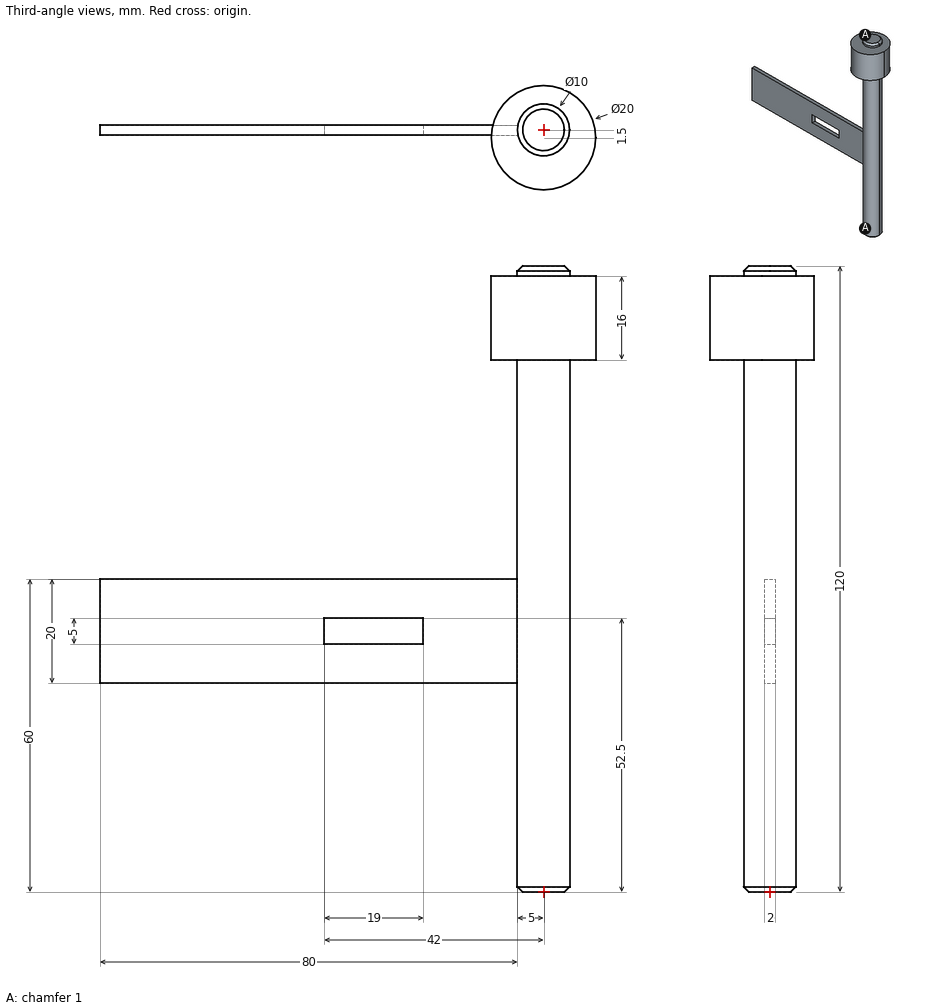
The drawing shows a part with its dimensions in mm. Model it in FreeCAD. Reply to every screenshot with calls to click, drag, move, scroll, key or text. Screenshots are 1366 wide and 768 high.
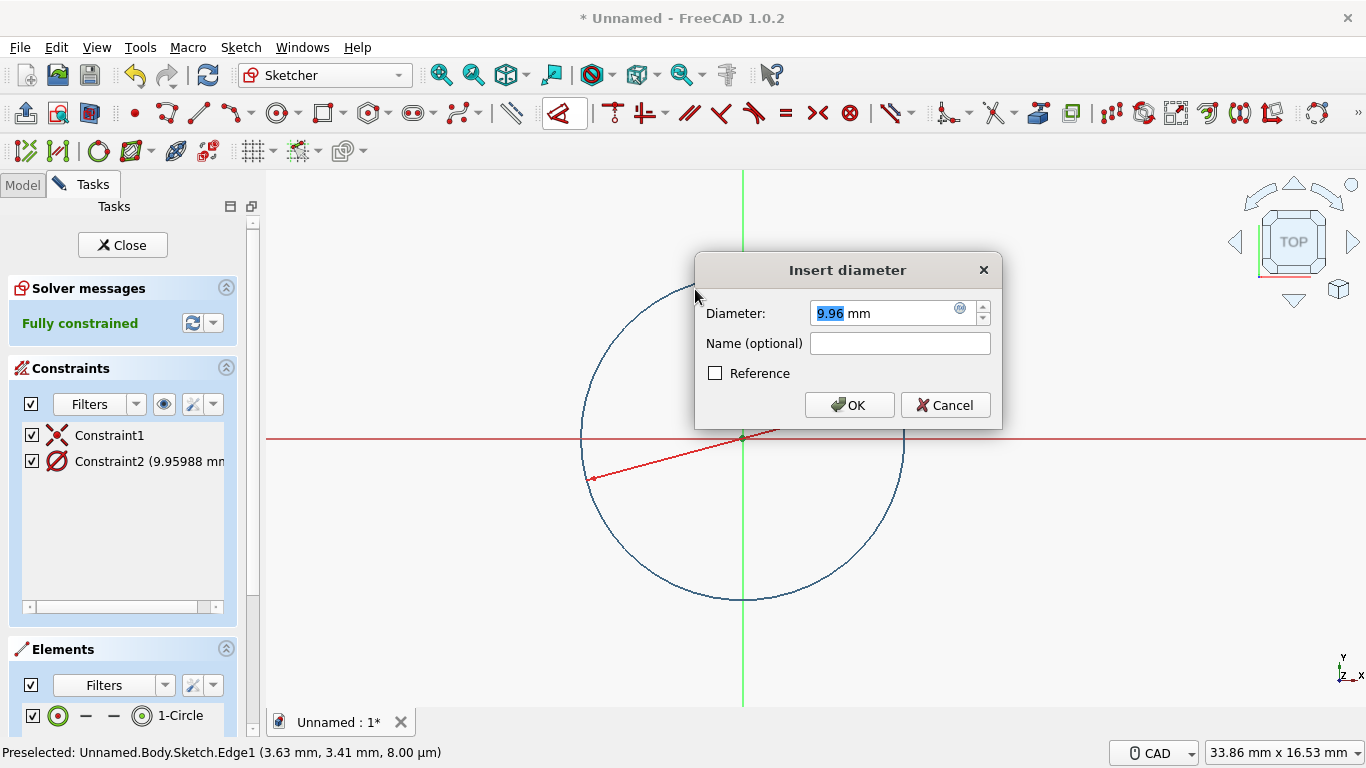
text(10)
key(Return)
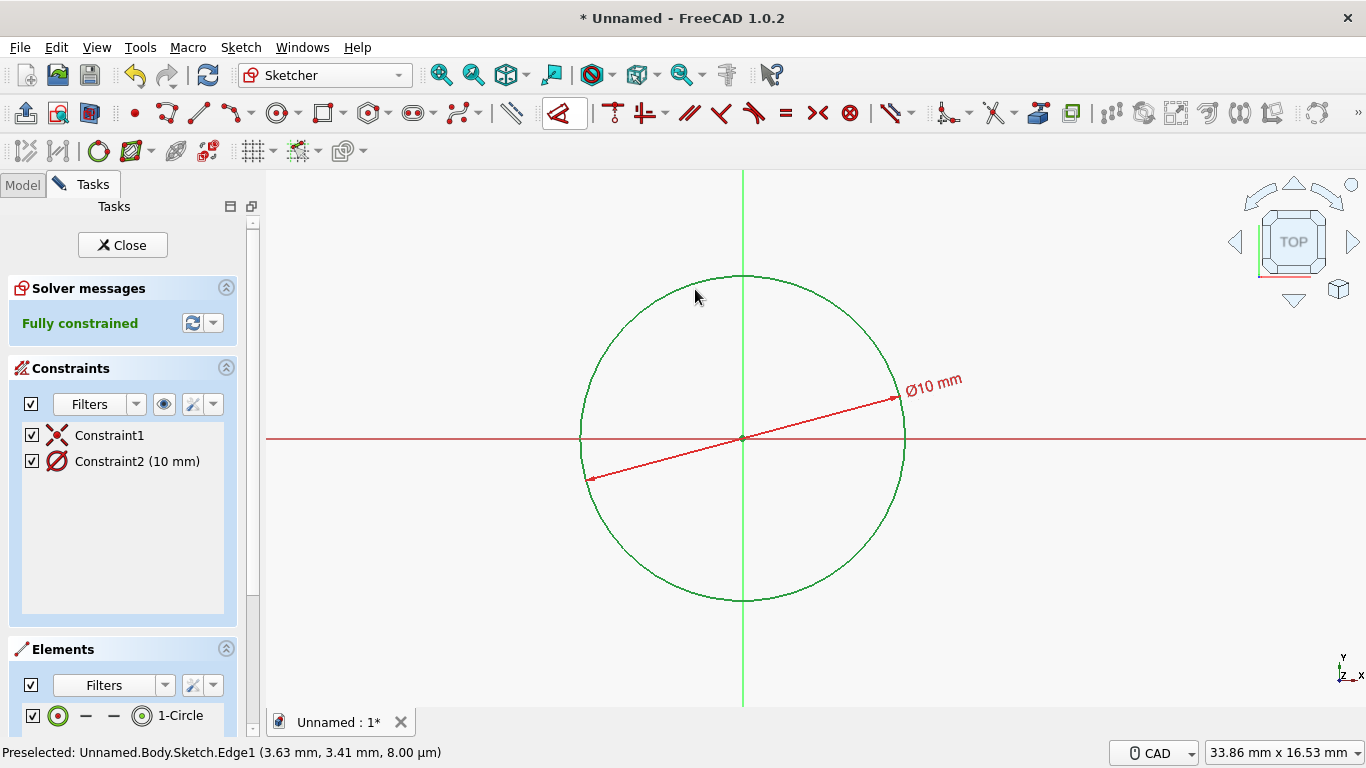
click(123, 245)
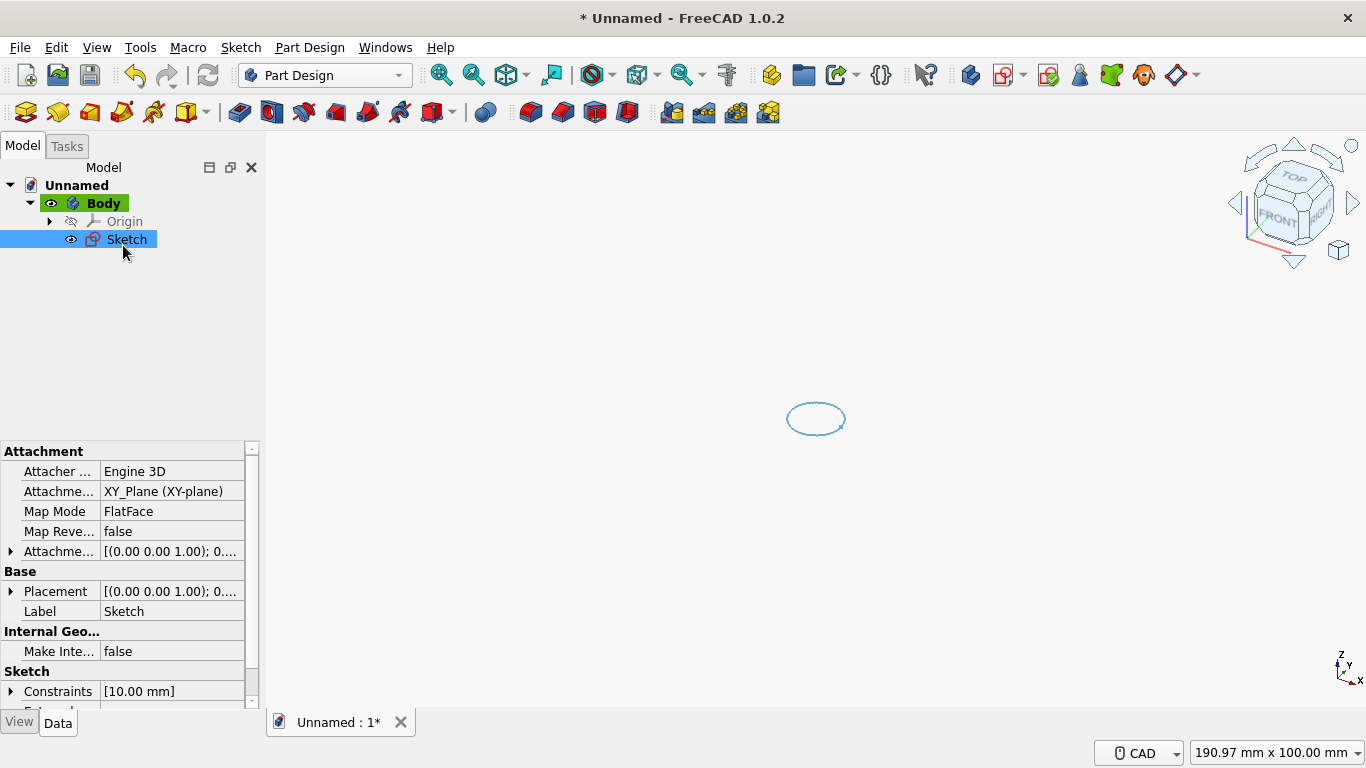
click(26, 112)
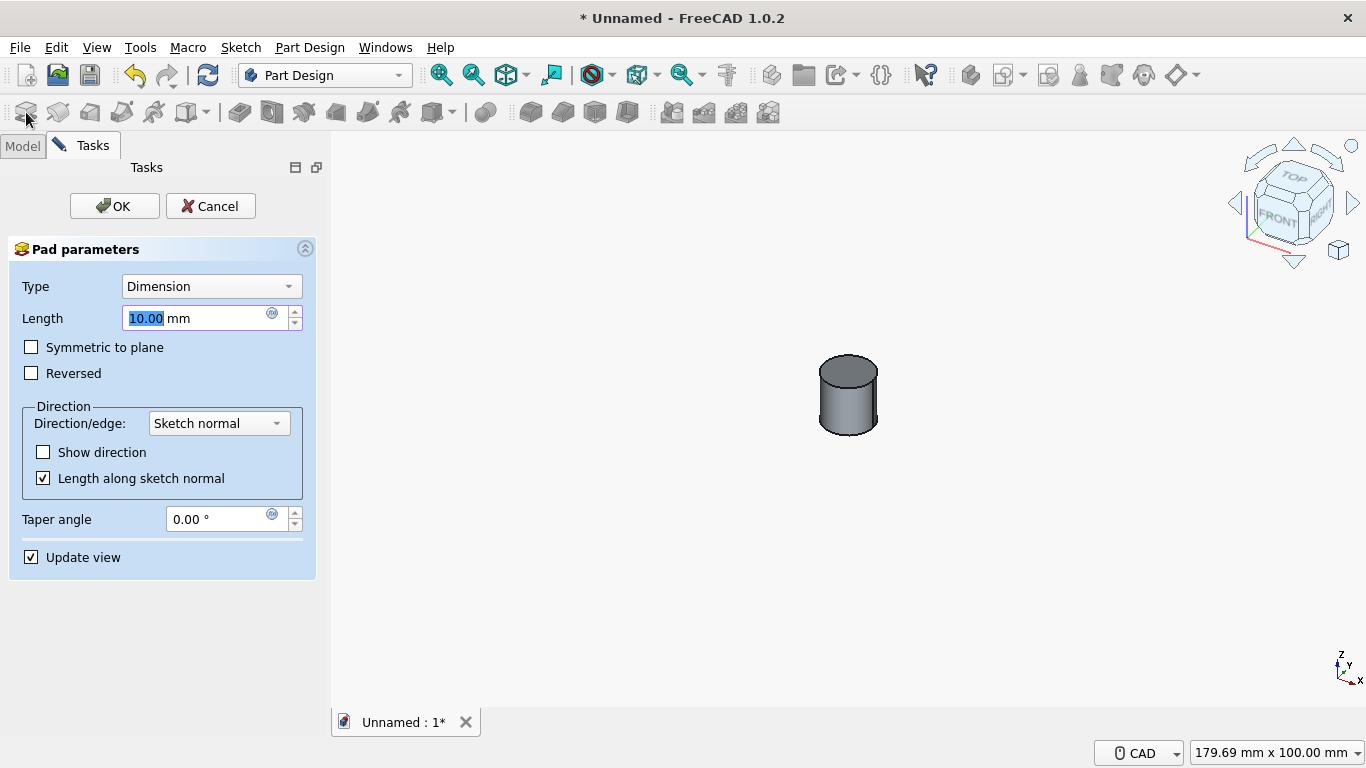
text(120)
key(Tab)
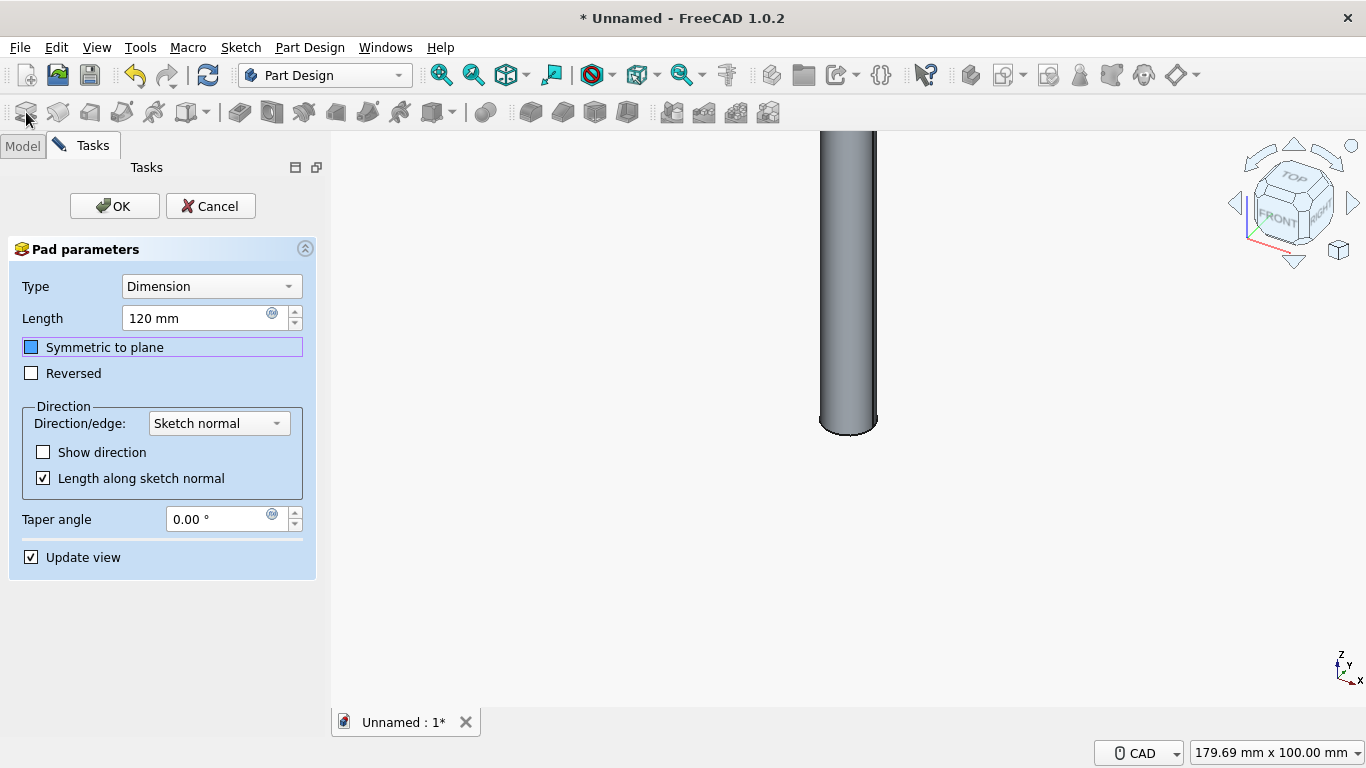
click(115, 206)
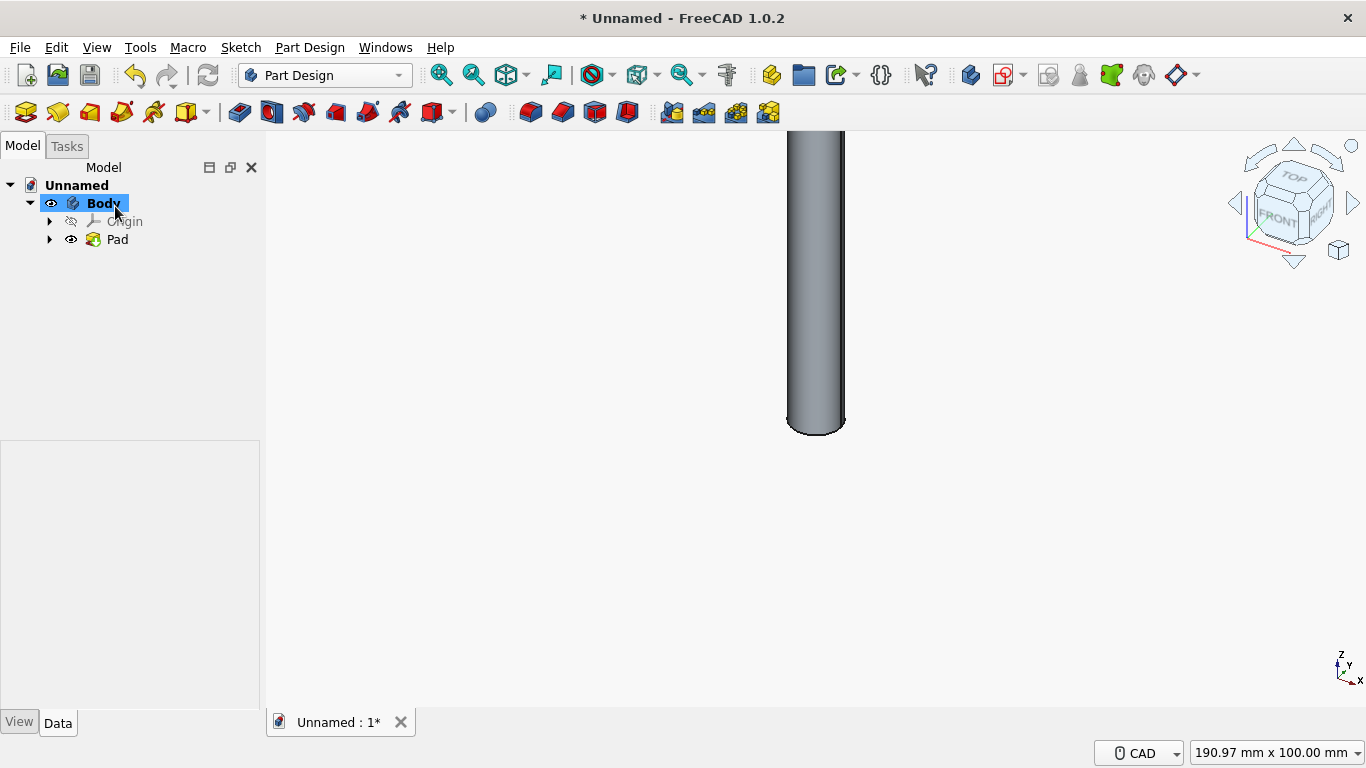
click(442, 76)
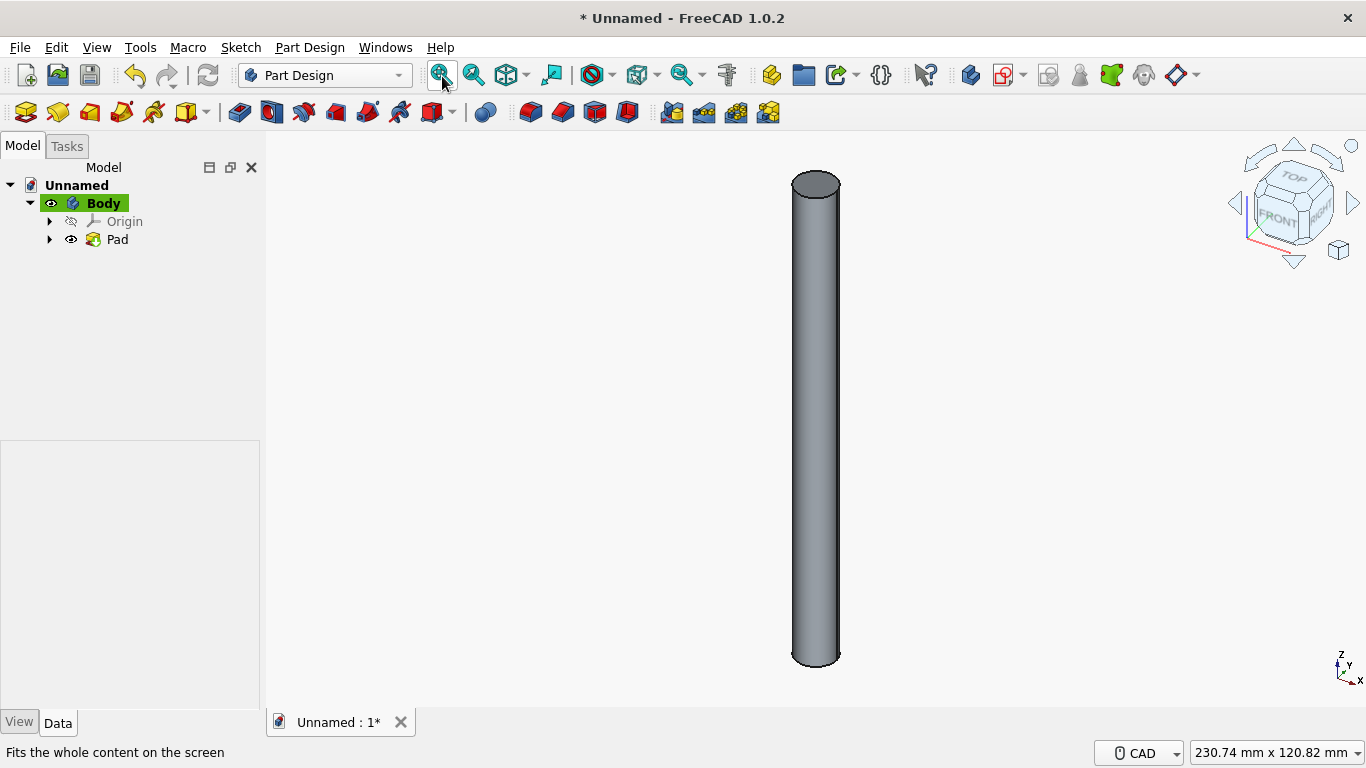
click(50, 221)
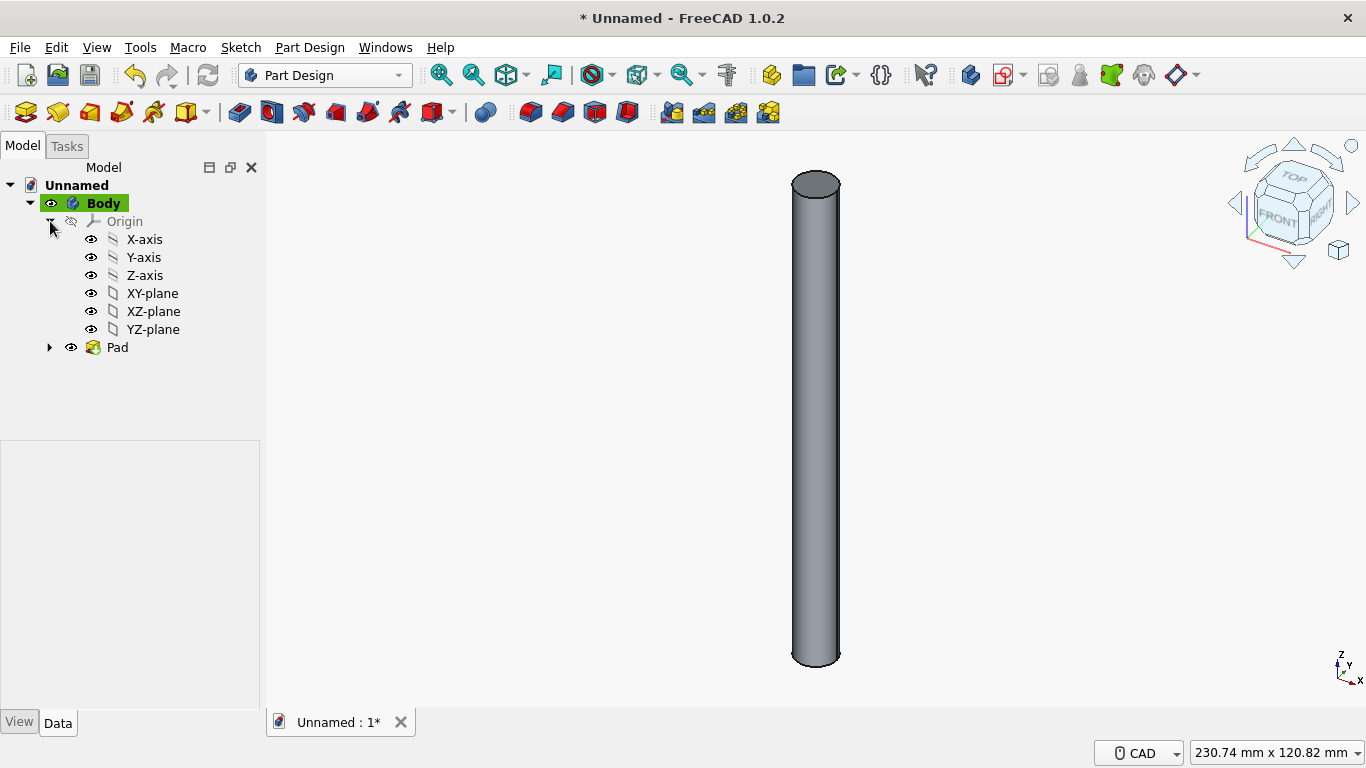
click(136, 293)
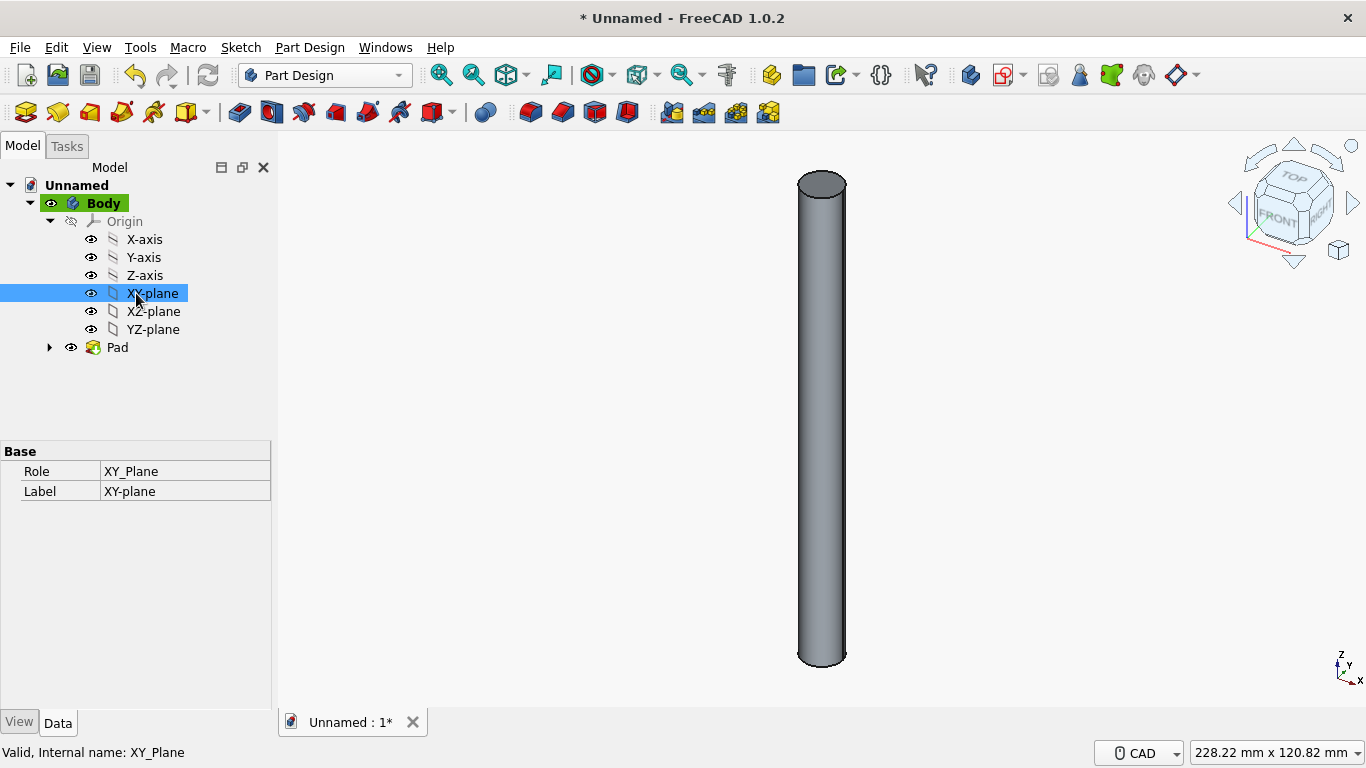
click(1176, 76)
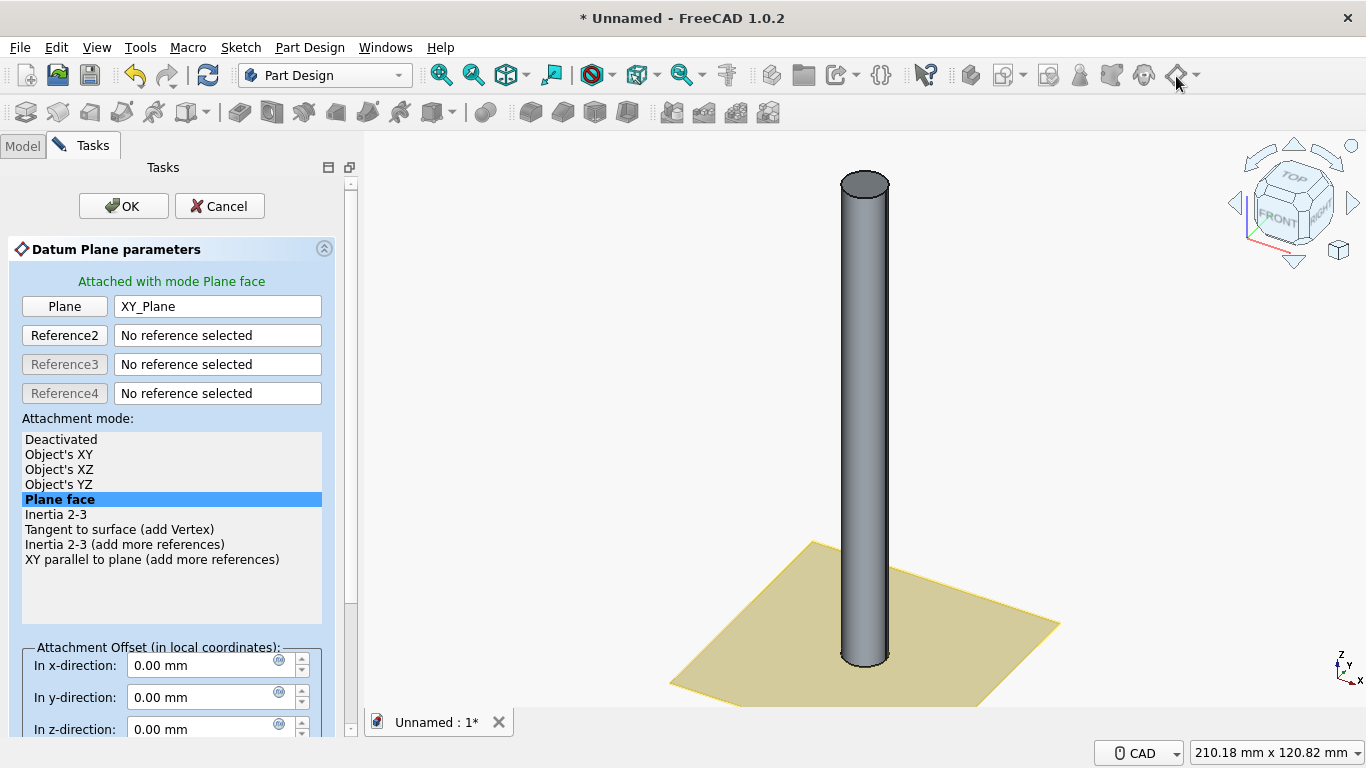
scroll(351, 456, down, 2)